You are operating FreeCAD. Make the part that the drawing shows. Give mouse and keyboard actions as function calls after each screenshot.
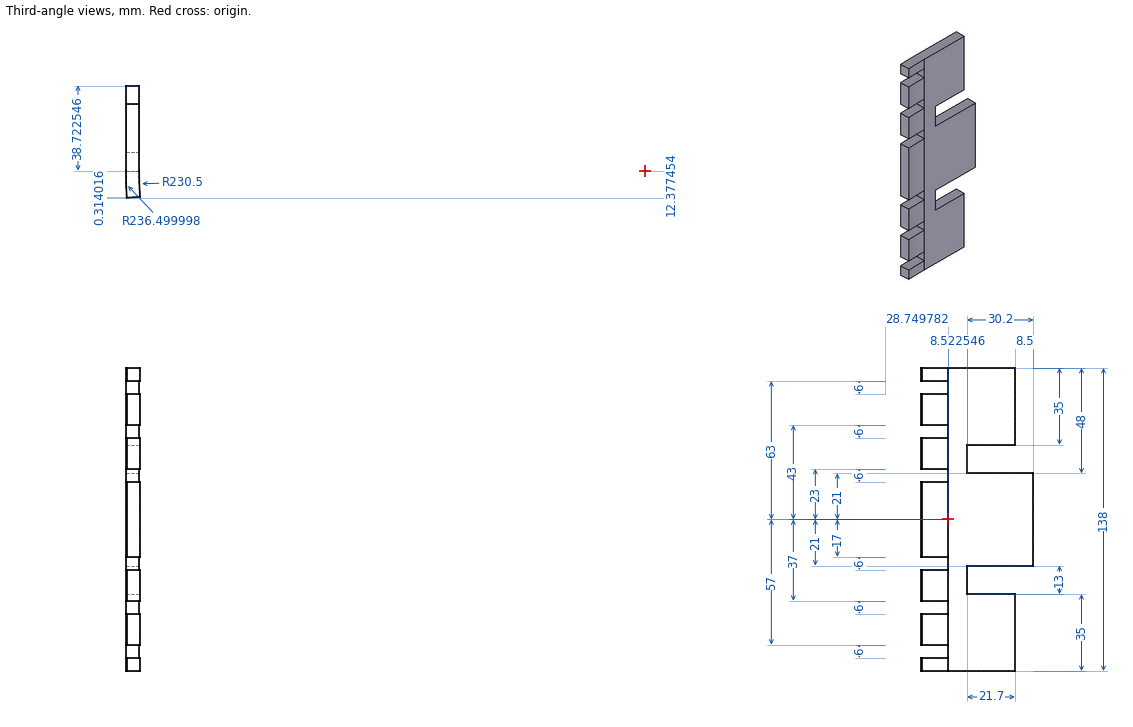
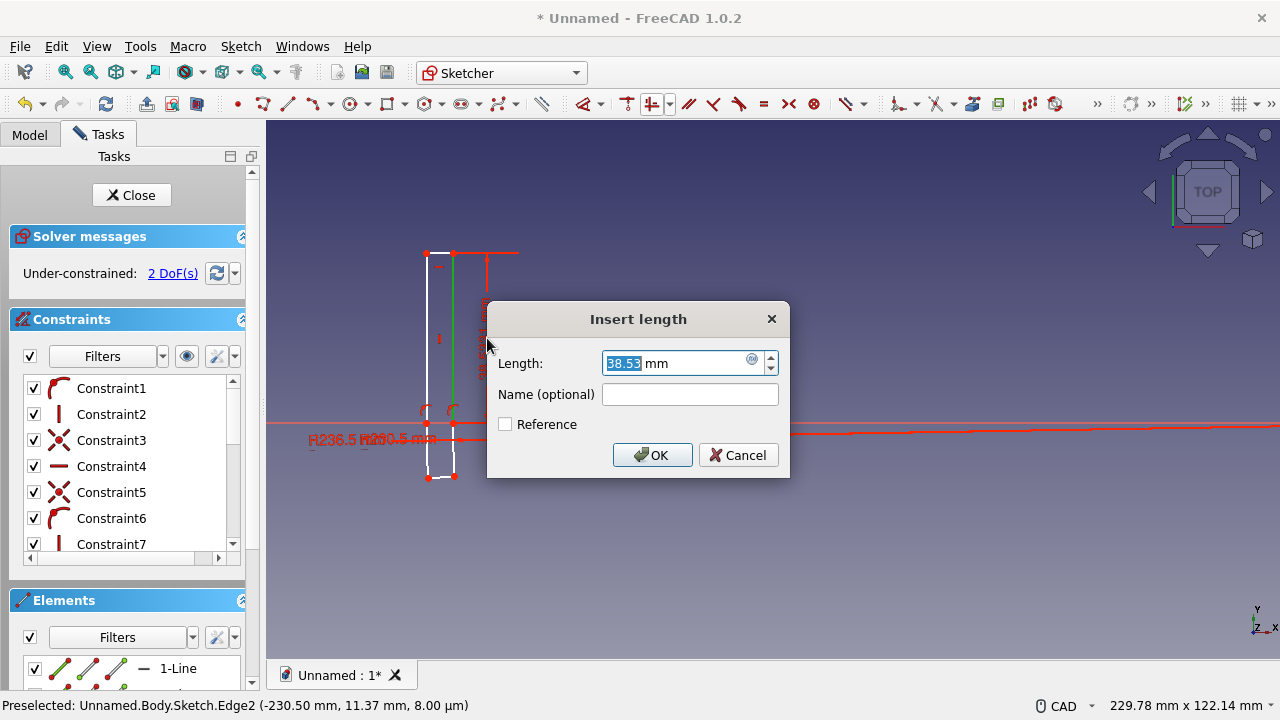
text(38.722546)
key(Return)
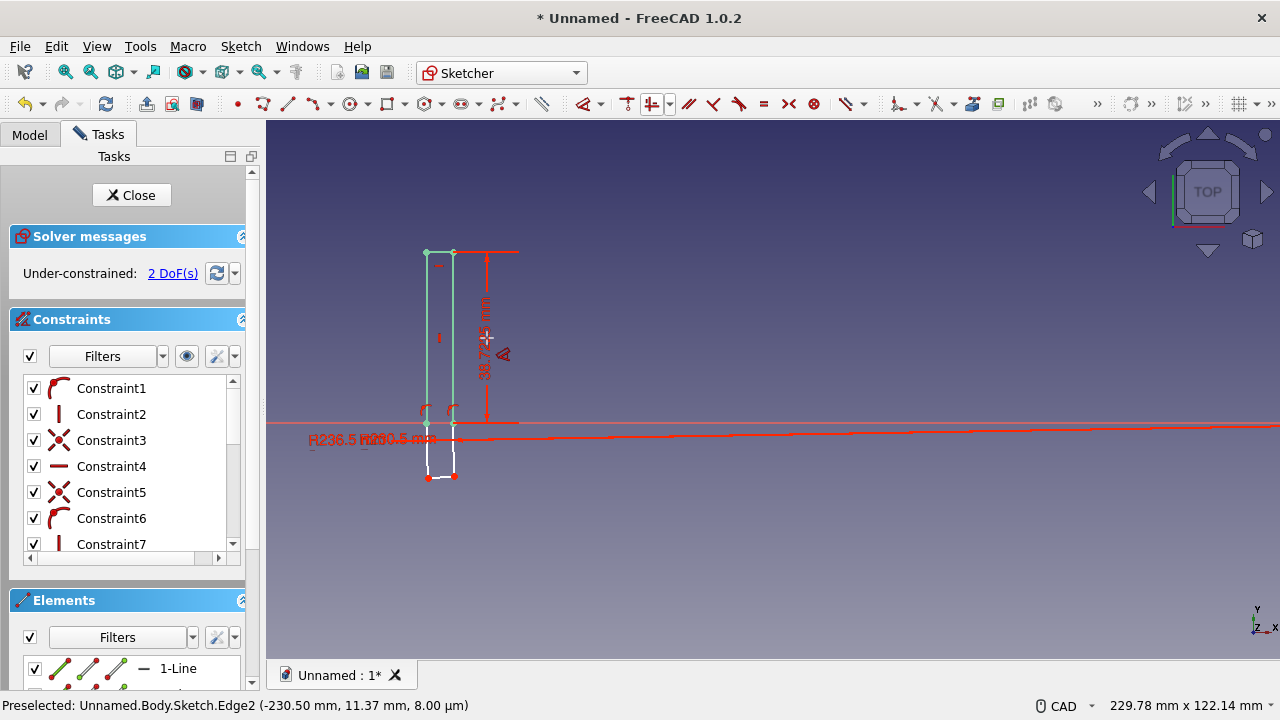
scroll(439, 478, up, 17)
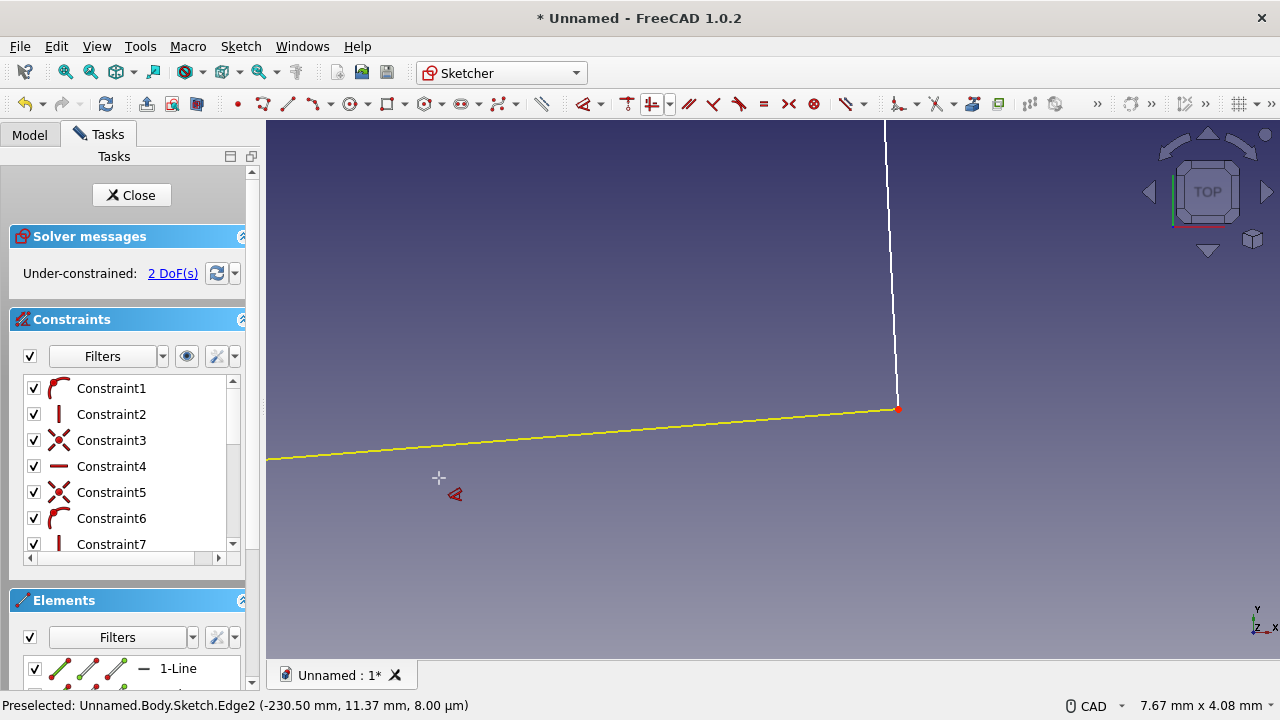
click(424, 447)
click(932, 441)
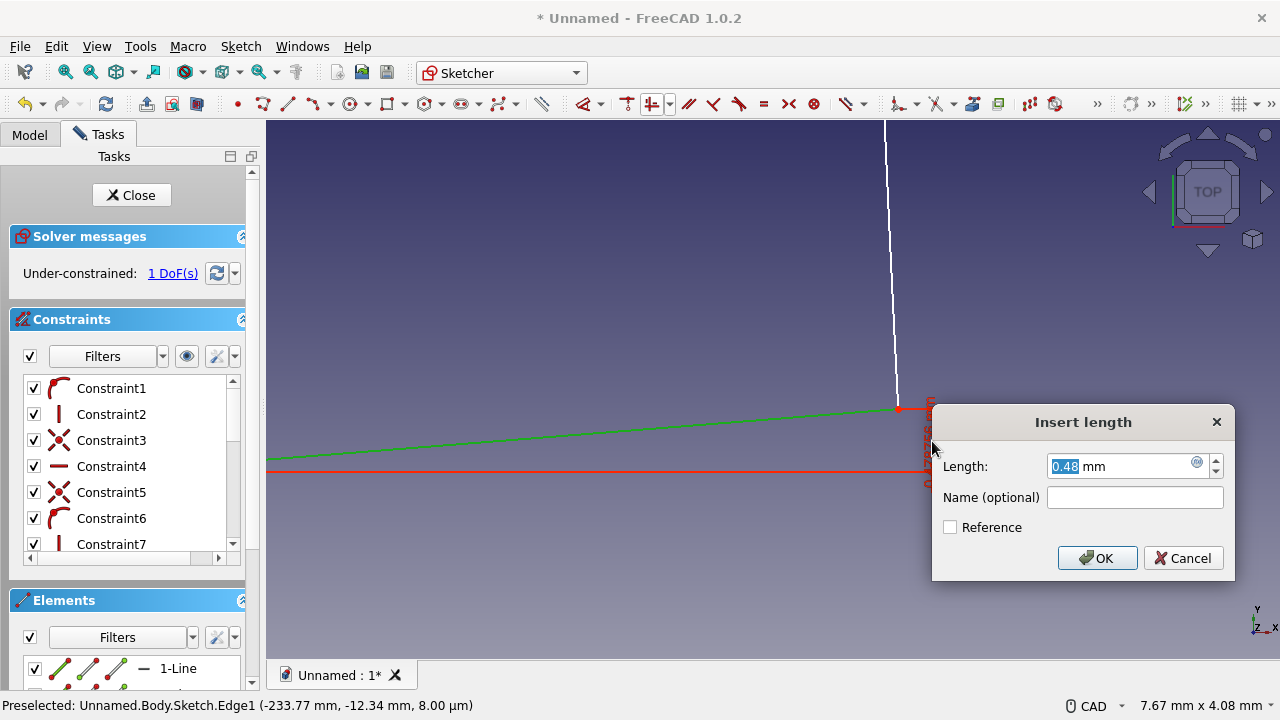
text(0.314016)
key(Return)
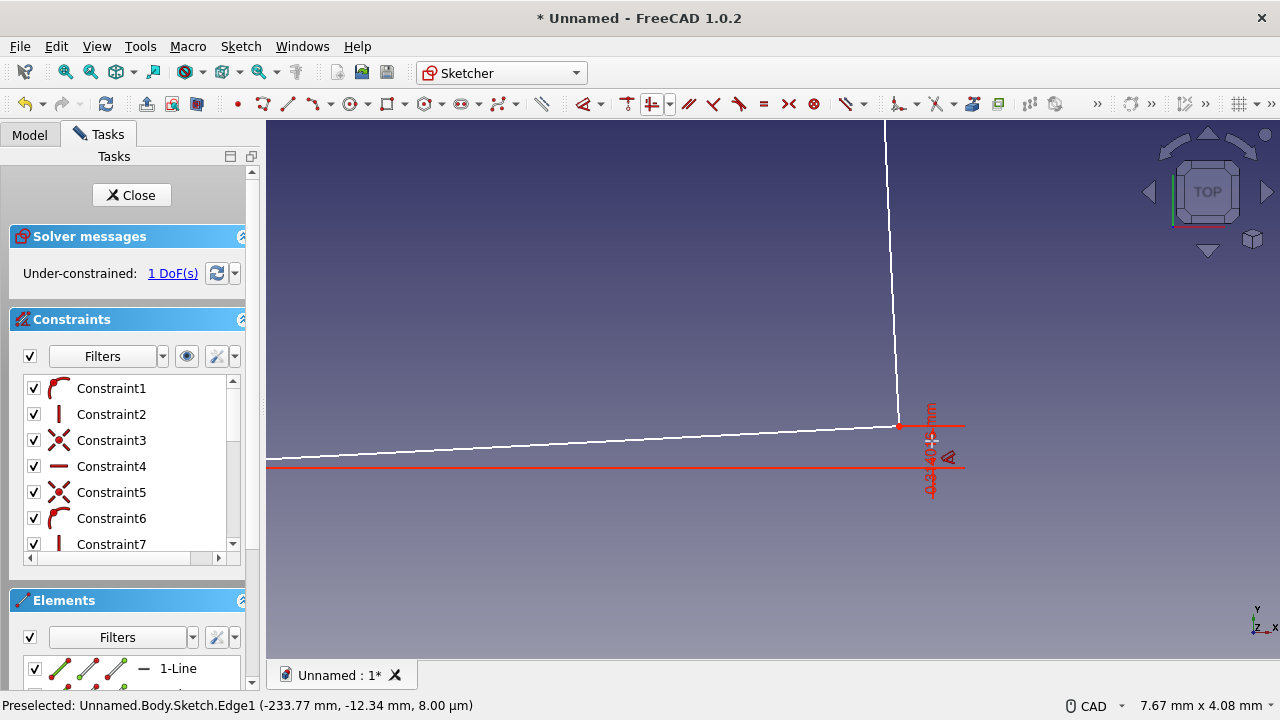
scroll(716, 563, down, 15)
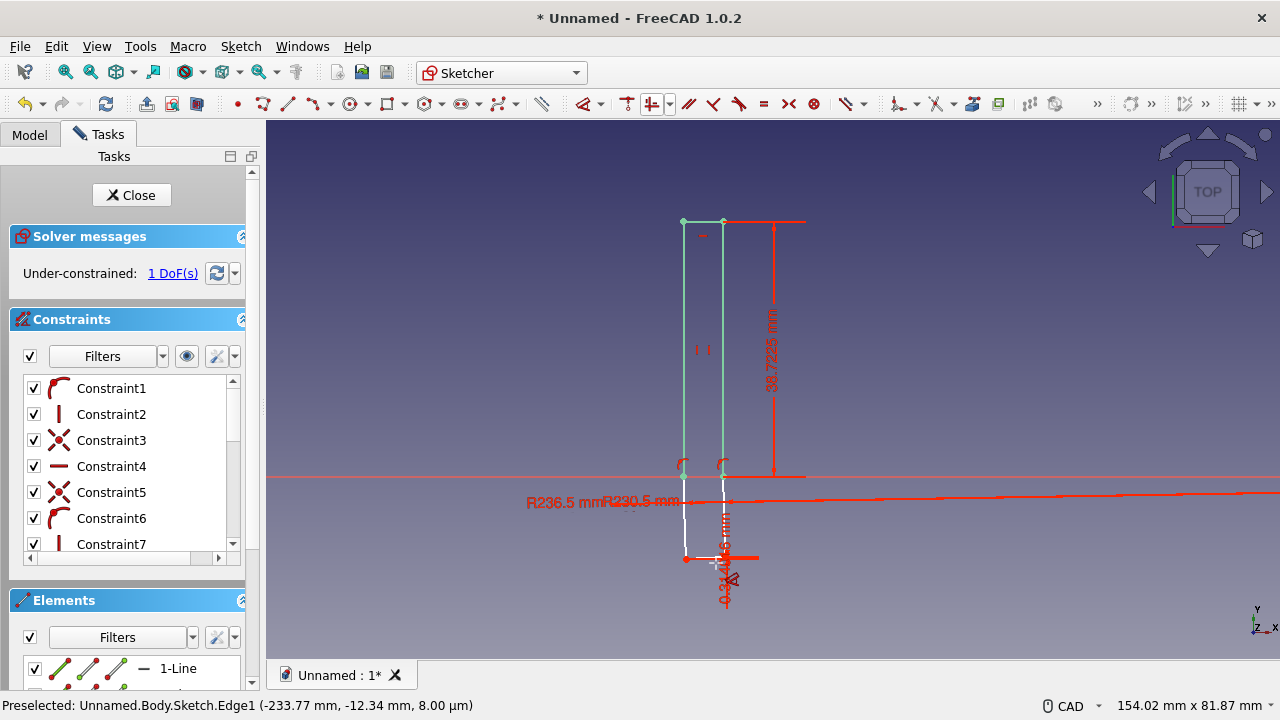
scroll(686, 559, up, 14)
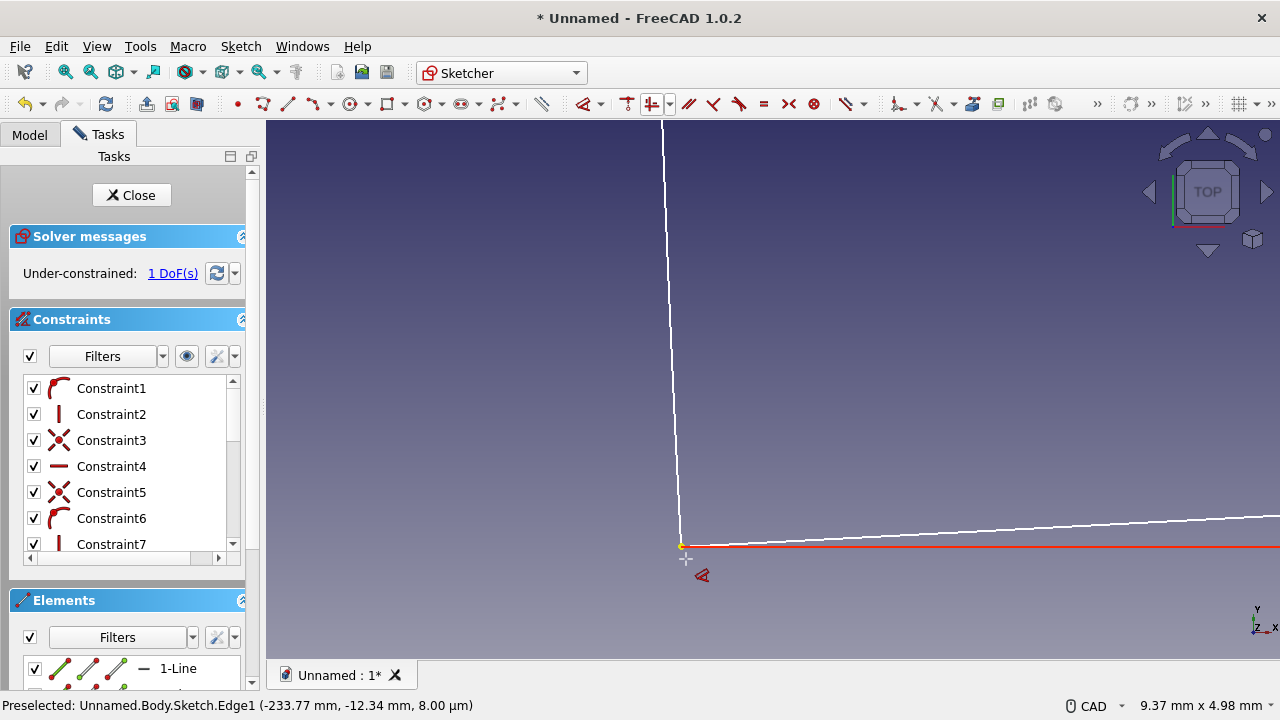
click(681, 547)
click(647, 347)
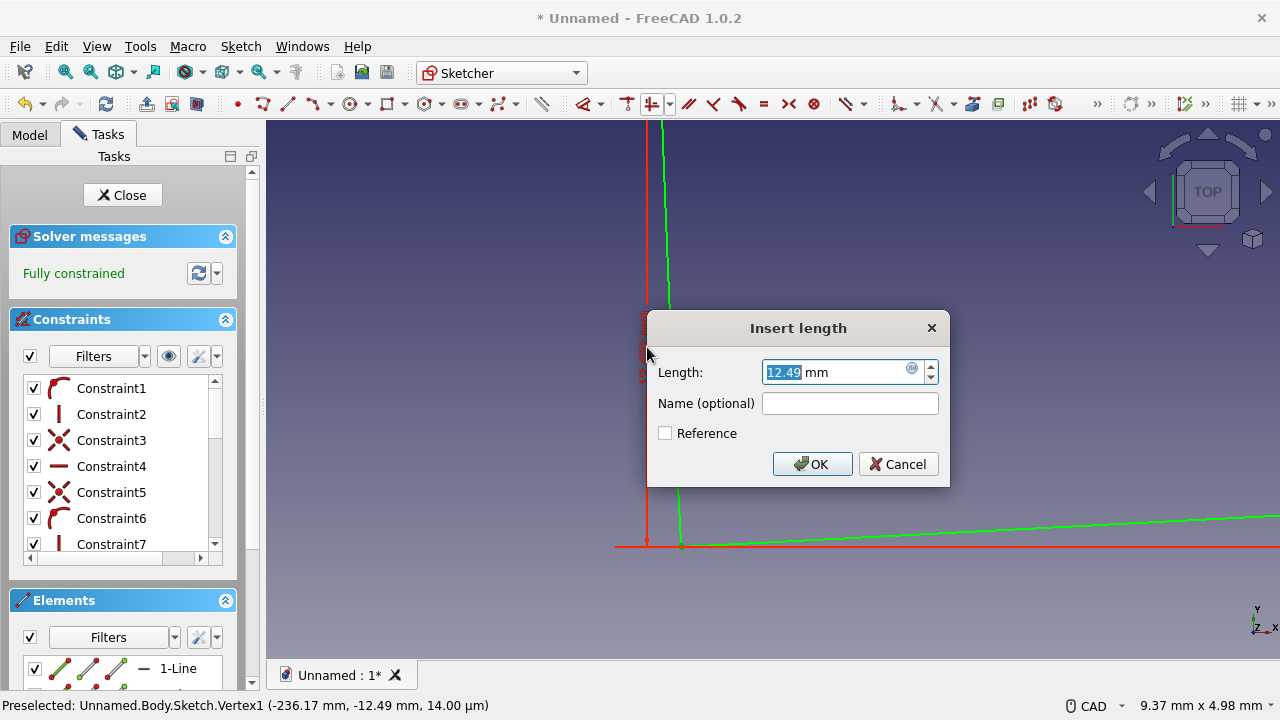
text(12.377454)
key(Return)
key(Escape)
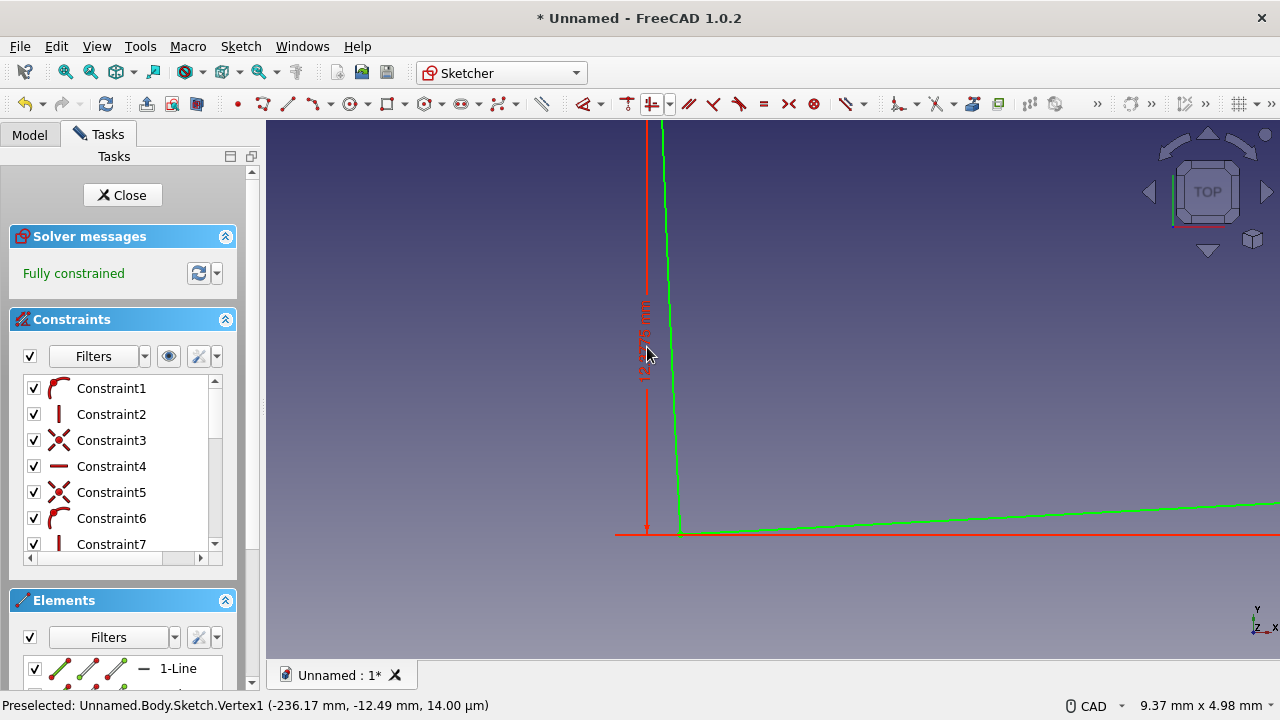
click(123, 195)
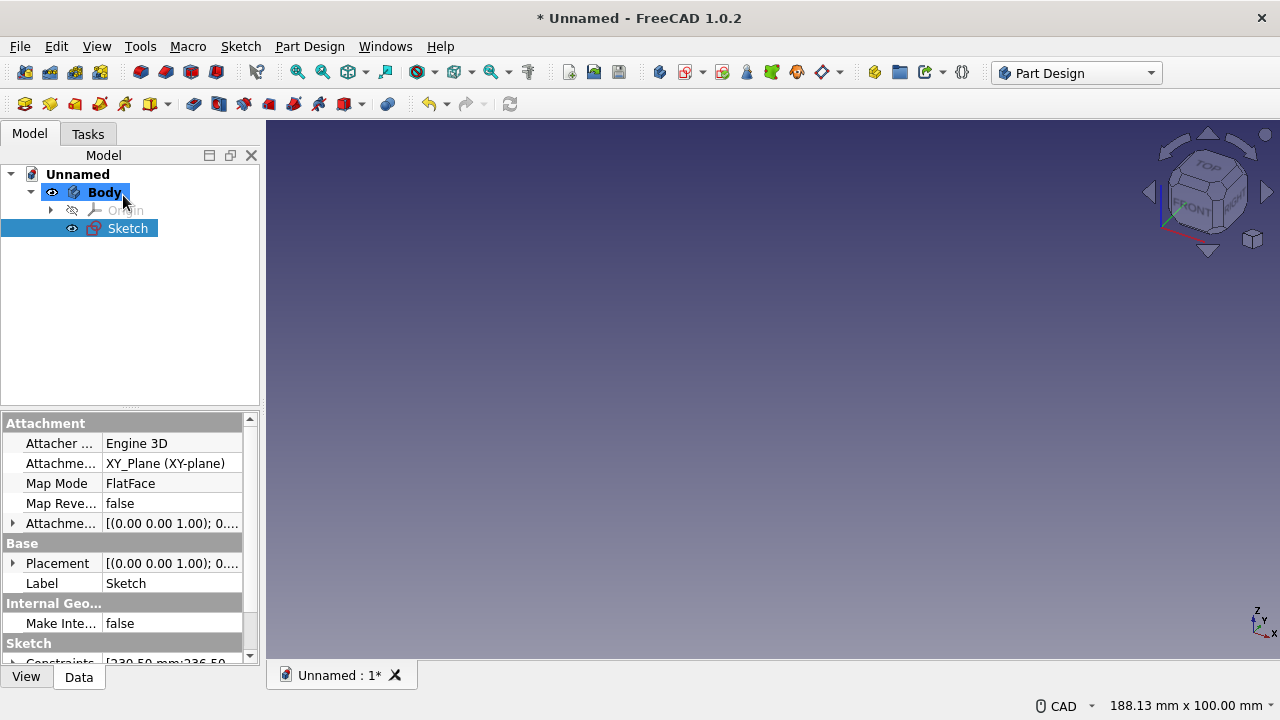
click(25, 104)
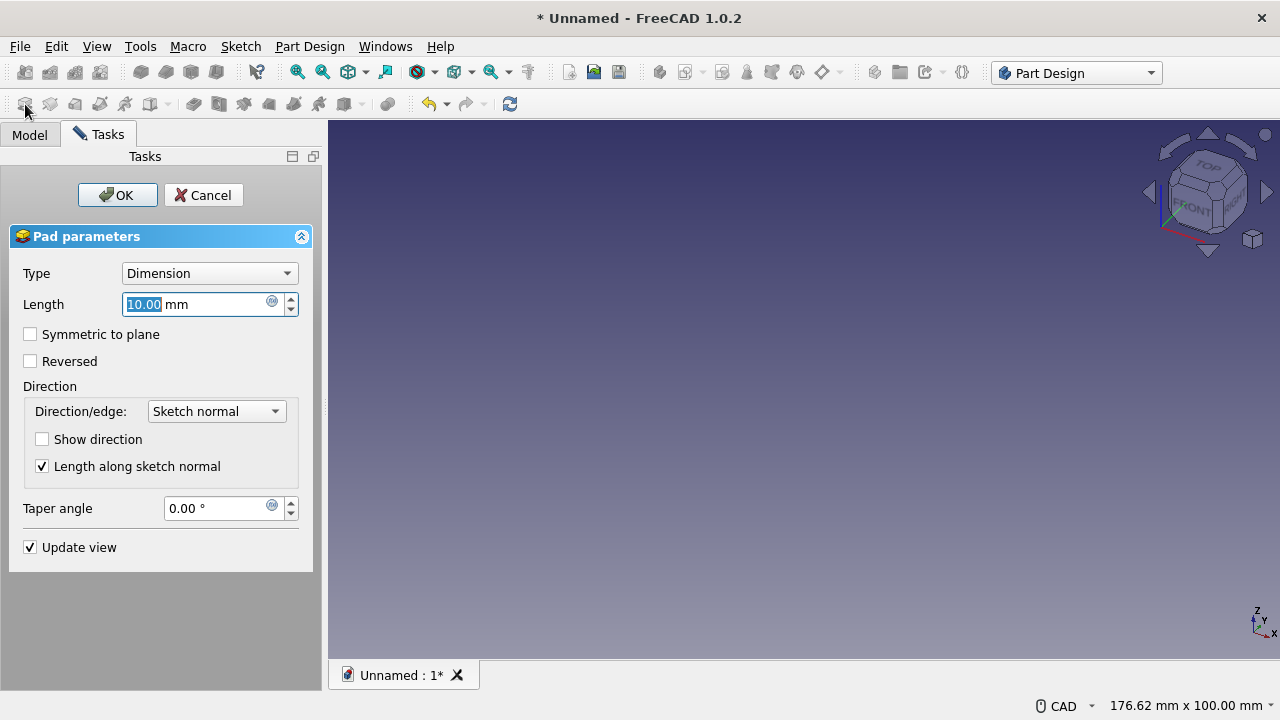
text(138)
key(Tab)